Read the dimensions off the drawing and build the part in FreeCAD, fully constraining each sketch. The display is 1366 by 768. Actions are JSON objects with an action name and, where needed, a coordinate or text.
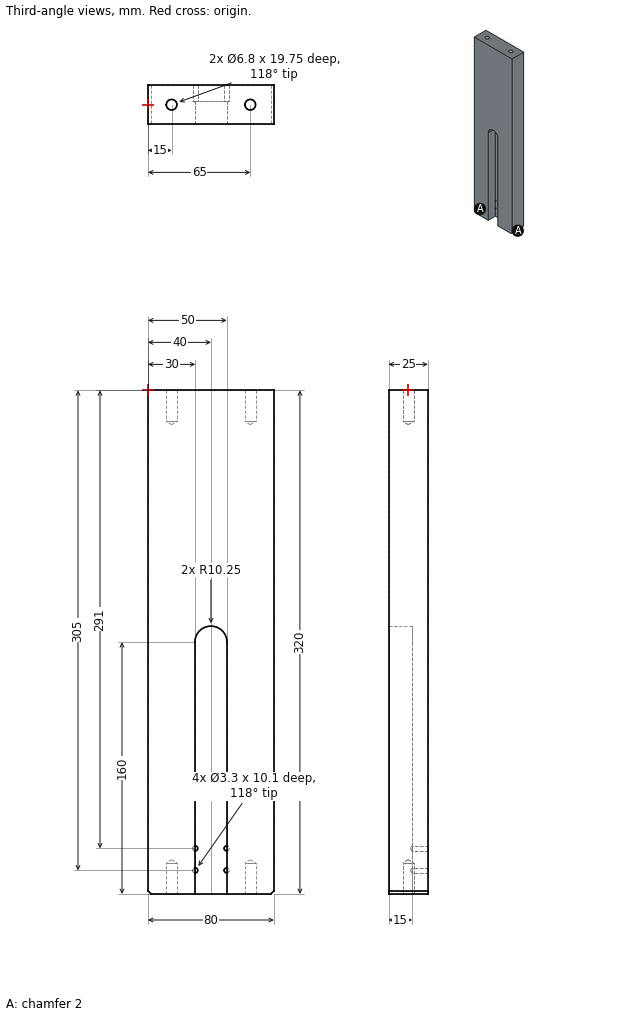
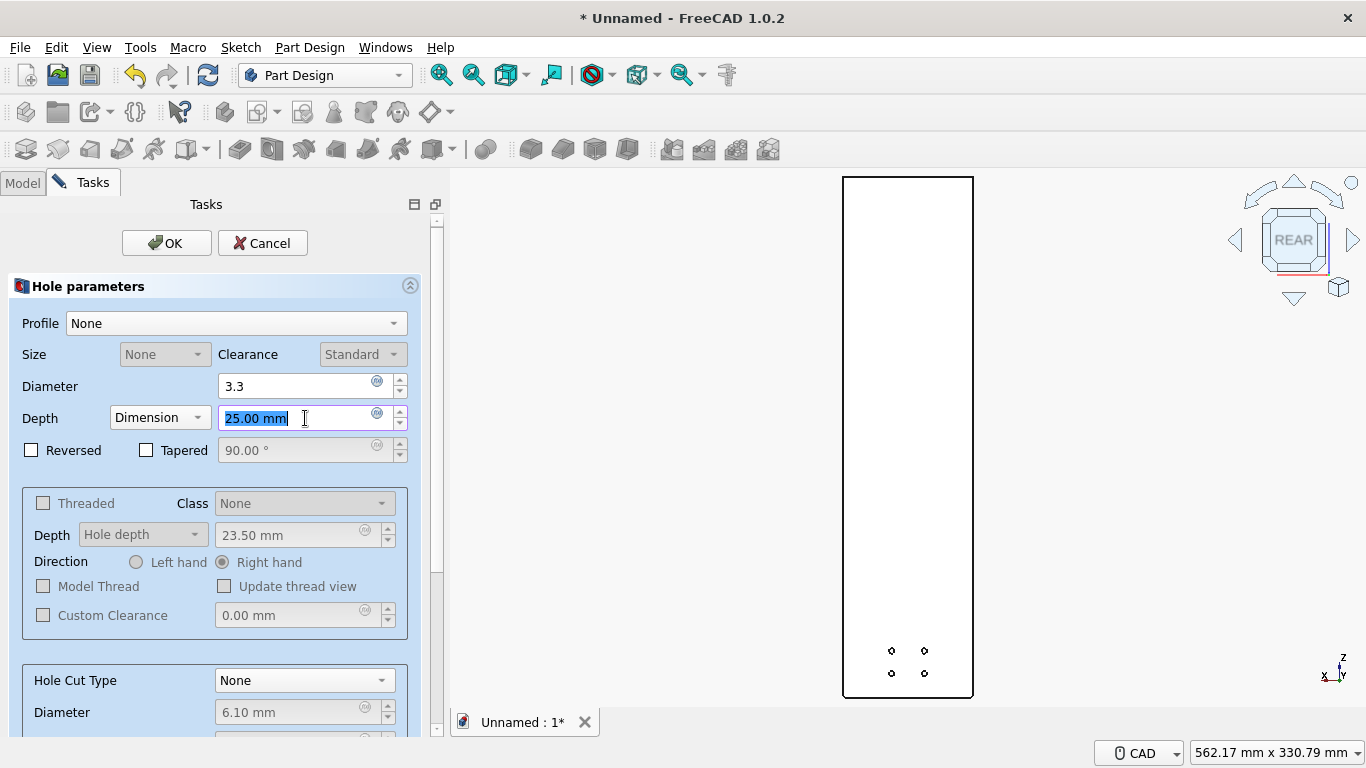
{"action": "type", "text": "10.1"}
{"action": "key", "text": "Tab"}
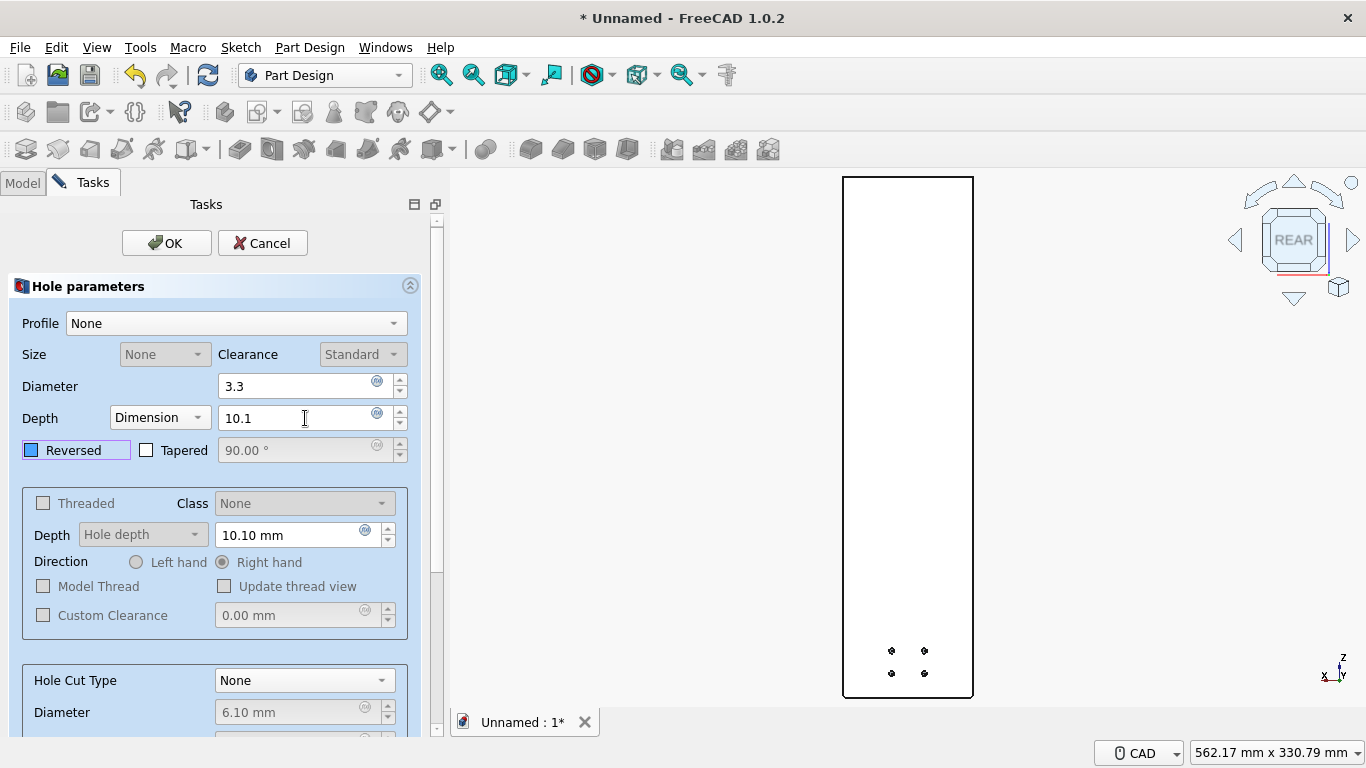
{"action": "left_click", "coordinate": [167, 243]}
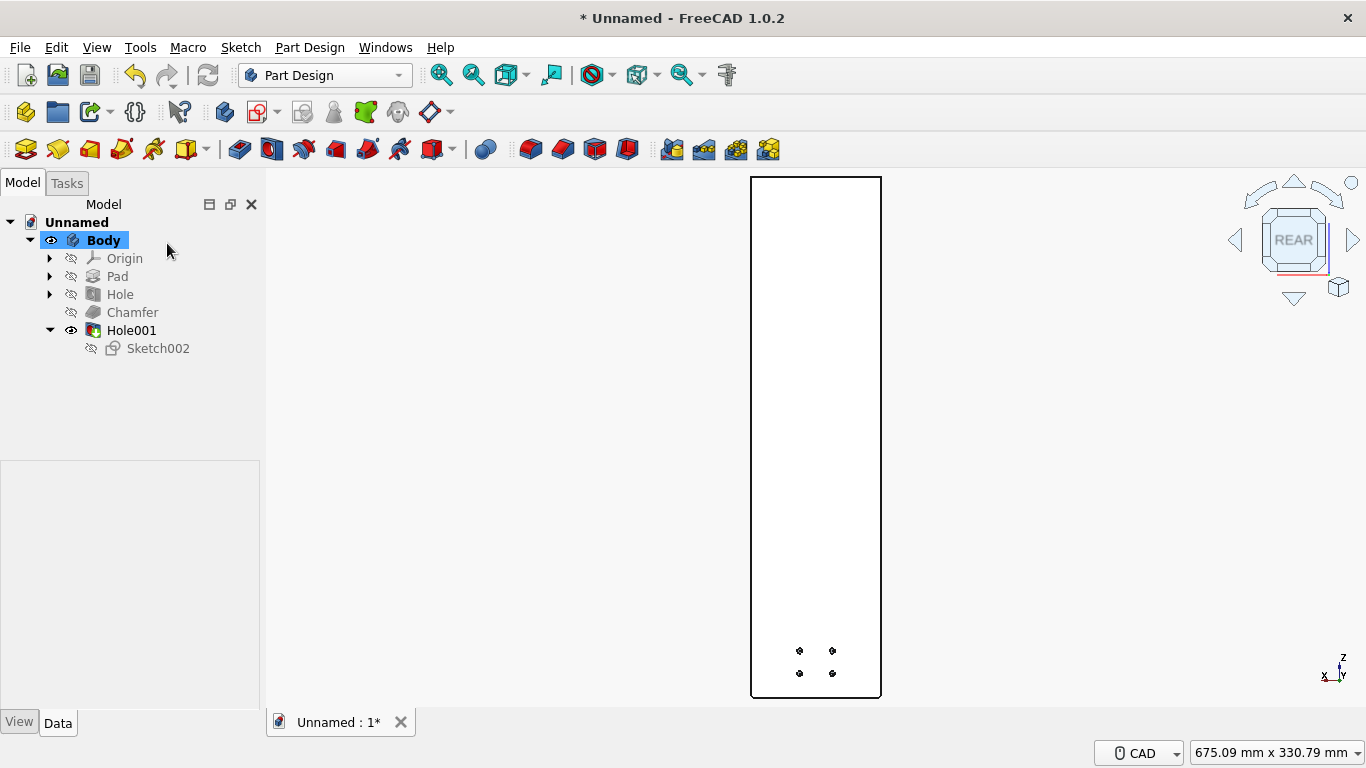
{"action": "key", "text": "5"}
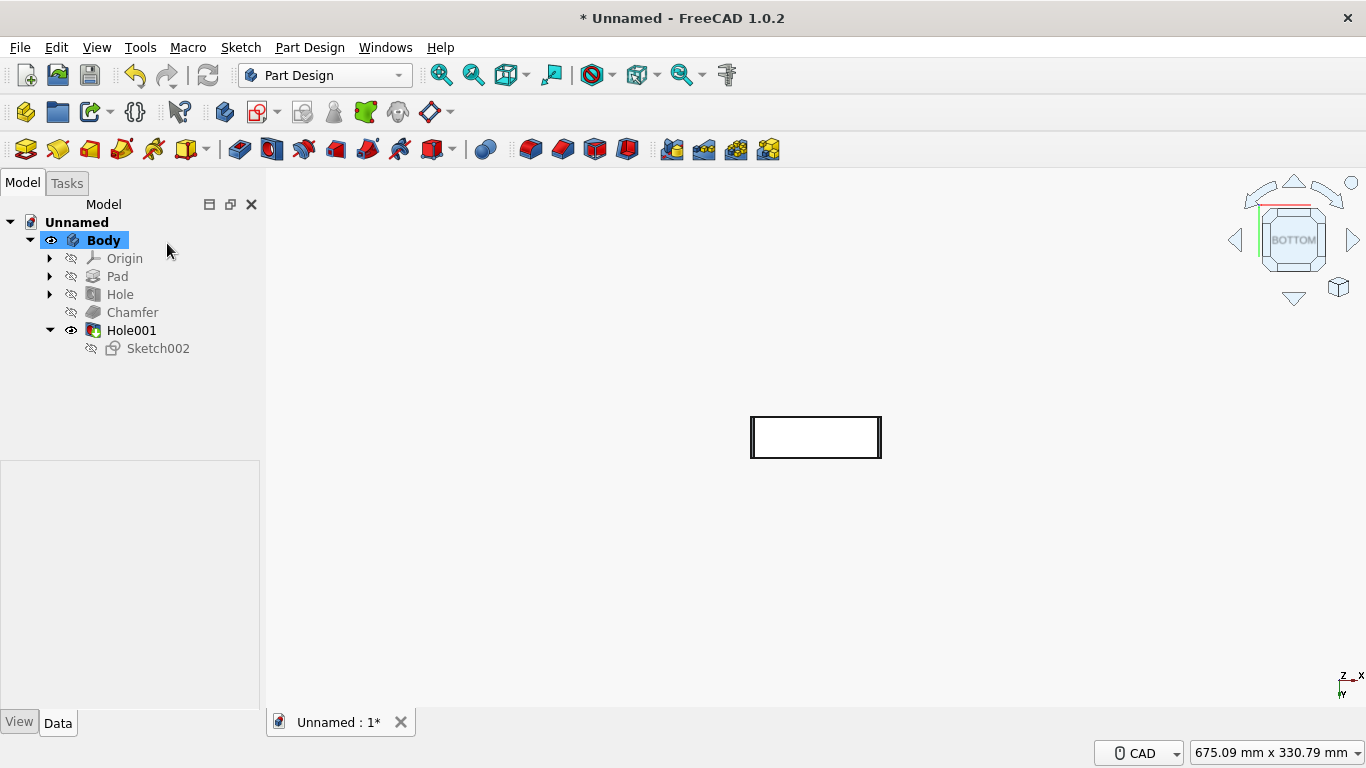
{"action": "left_click", "coordinate": [442, 76]}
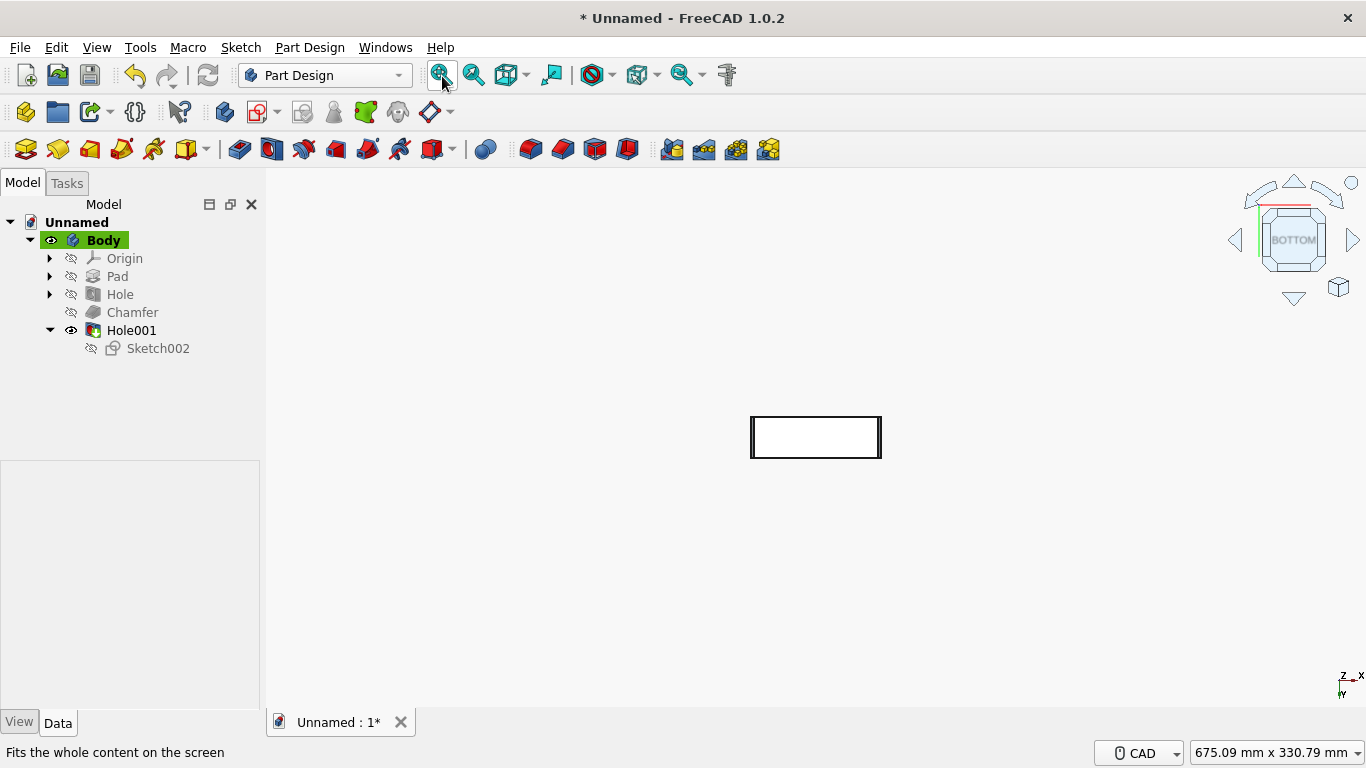
{"action": "left_click", "coordinate": [851, 436]}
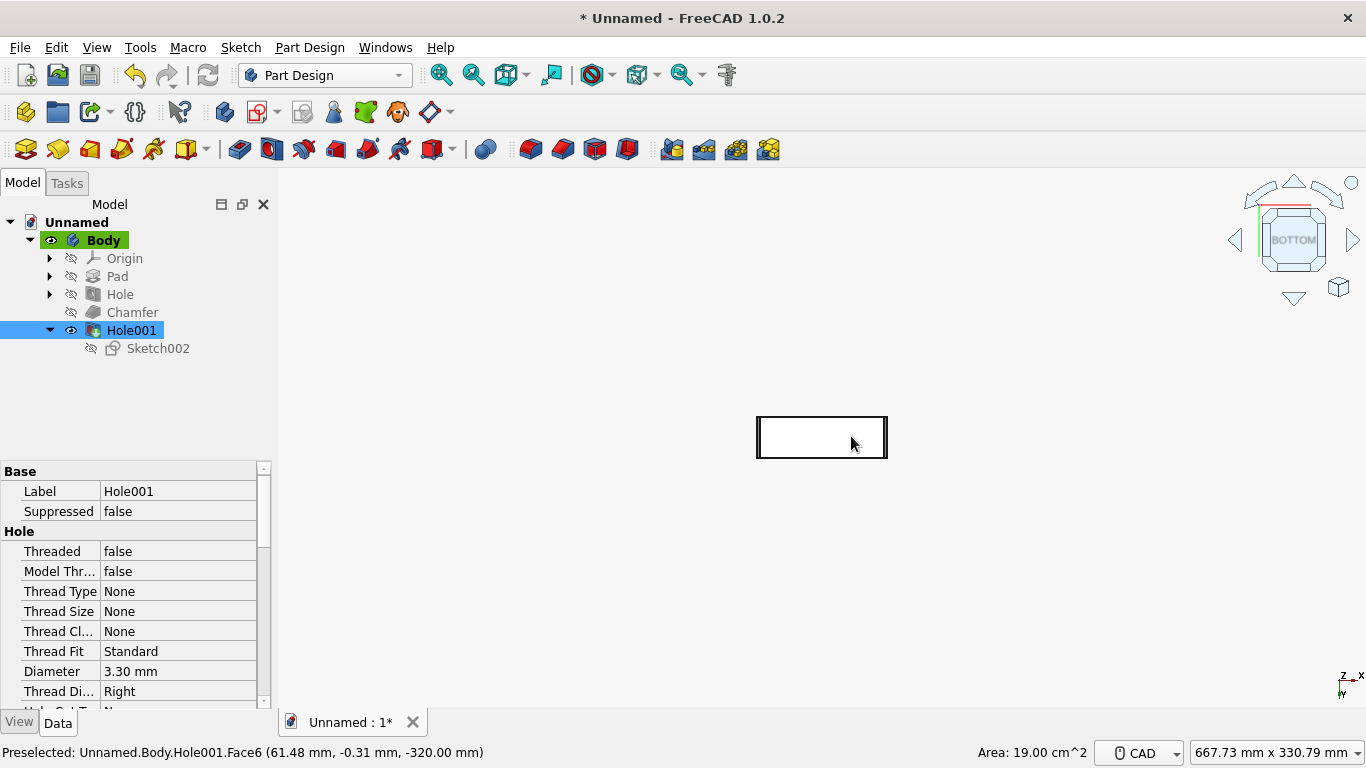
{"action": "left_click", "coordinate": [258, 112]}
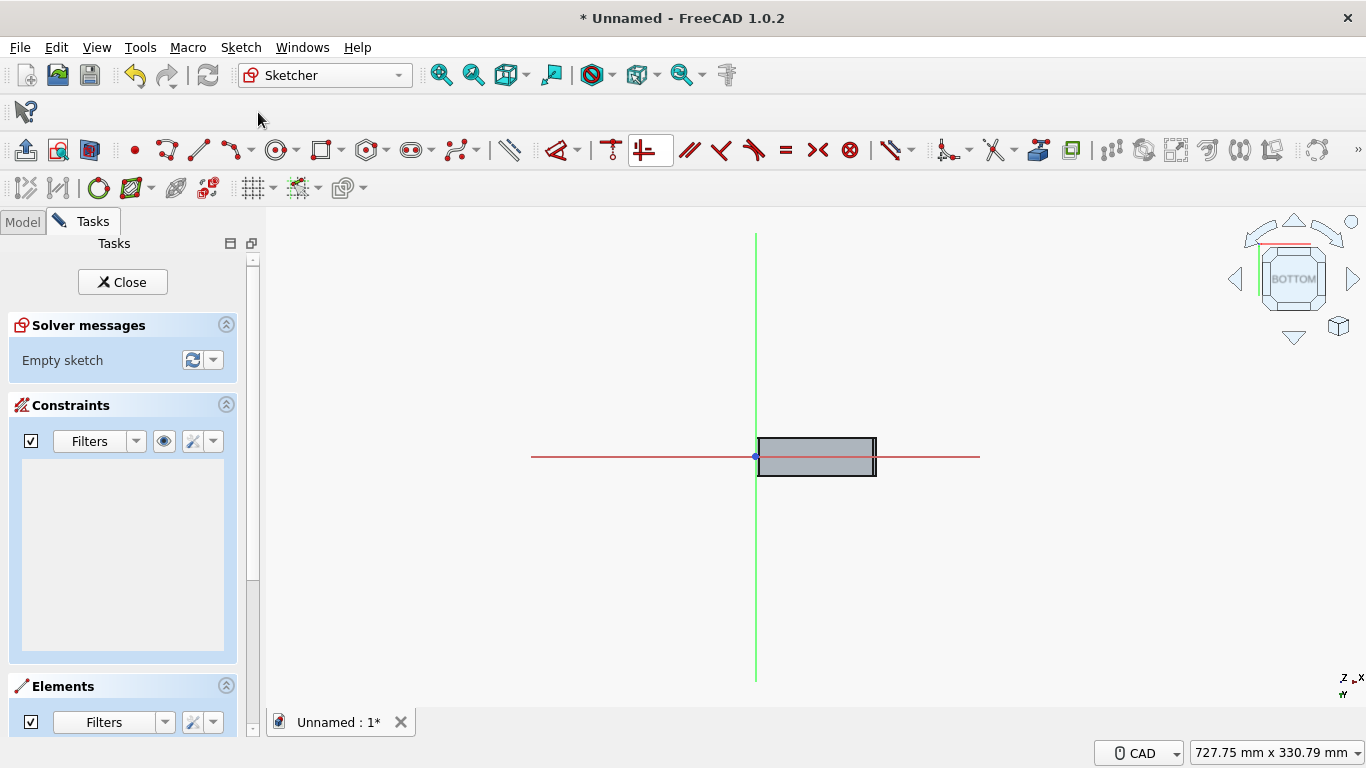
{"action": "scroll", "coordinate": [819, 457], "scroll_direction": "up", "scroll_amount": 9}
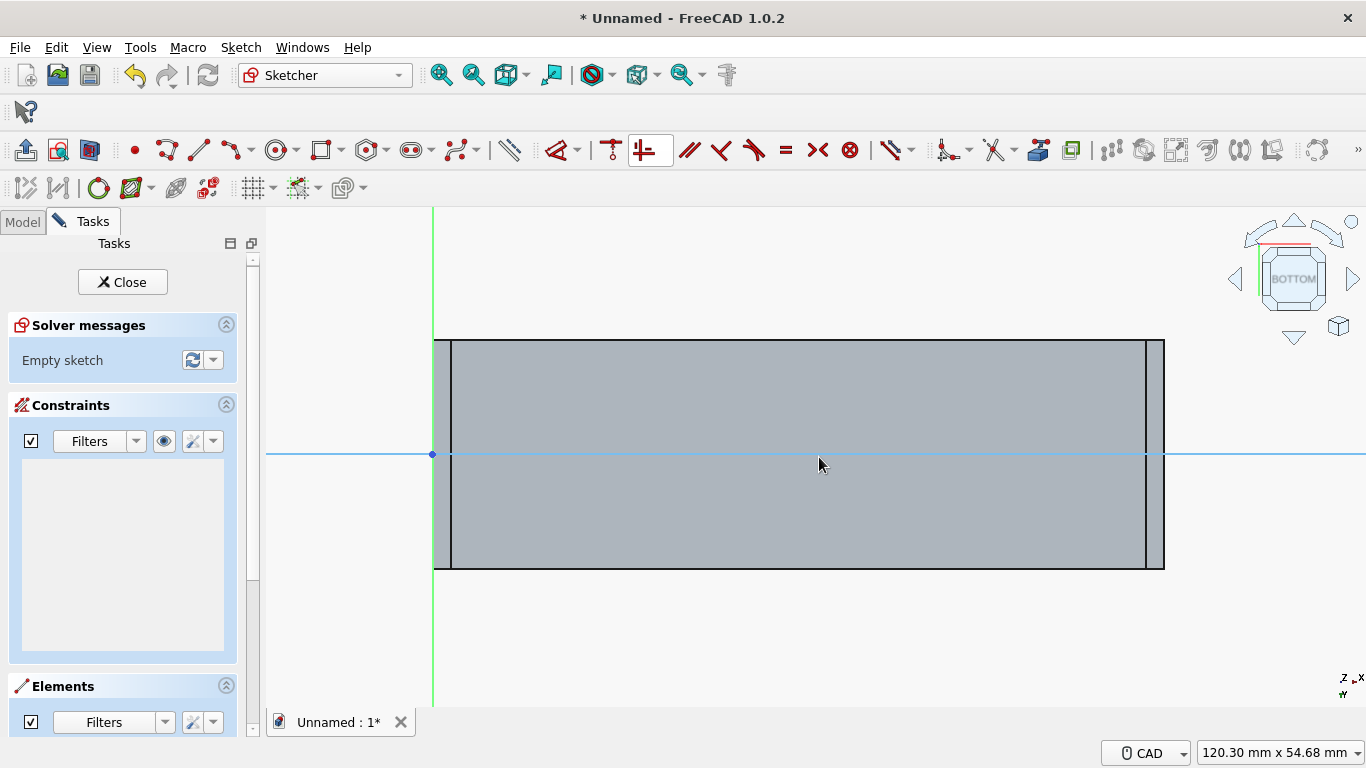
{"action": "key", "text": "g c"}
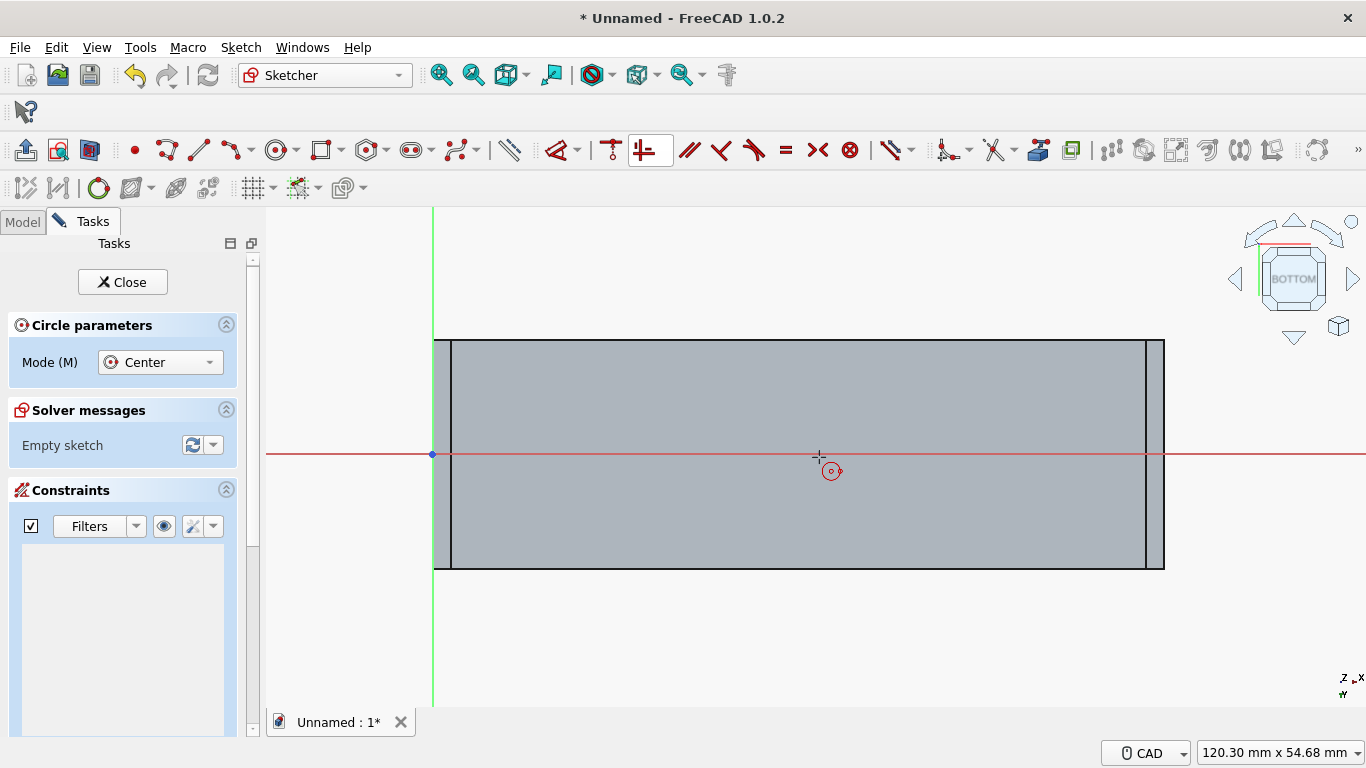
{"action": "left_click", "coordinate": [570, 454]}
{"action": "mouse_move", "coordinate": [592, 432]}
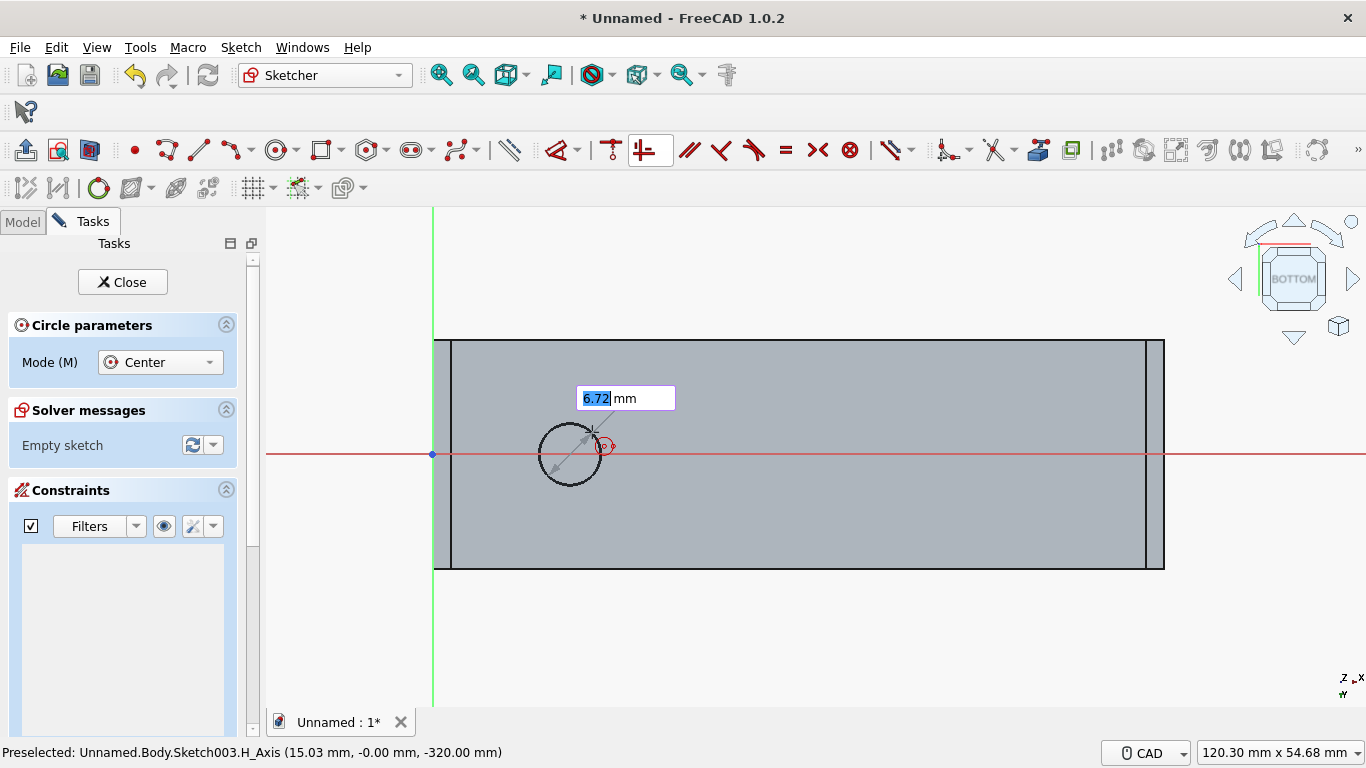
{"action": "type", "text": "6.8"}
{"action": "key", "text": "Return"}